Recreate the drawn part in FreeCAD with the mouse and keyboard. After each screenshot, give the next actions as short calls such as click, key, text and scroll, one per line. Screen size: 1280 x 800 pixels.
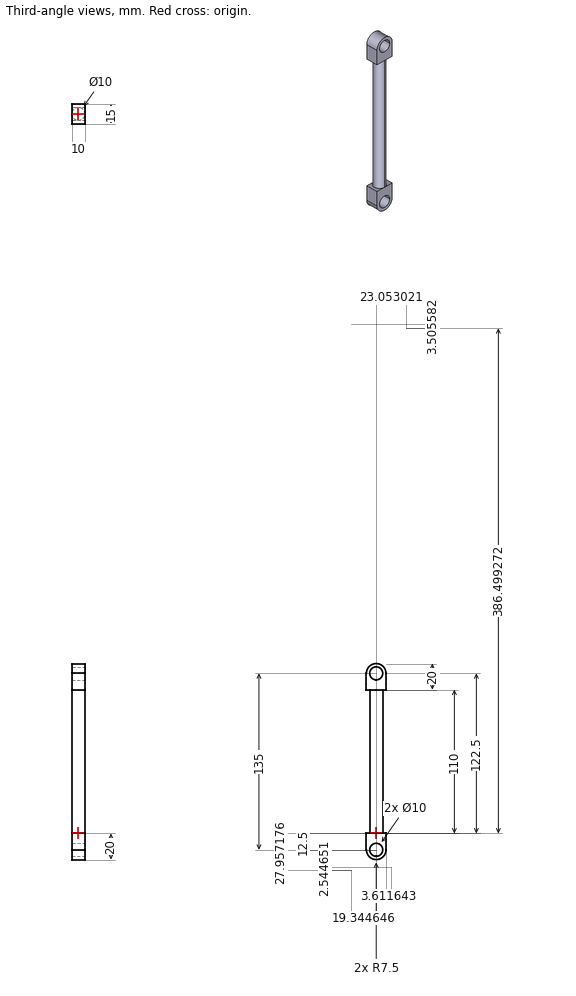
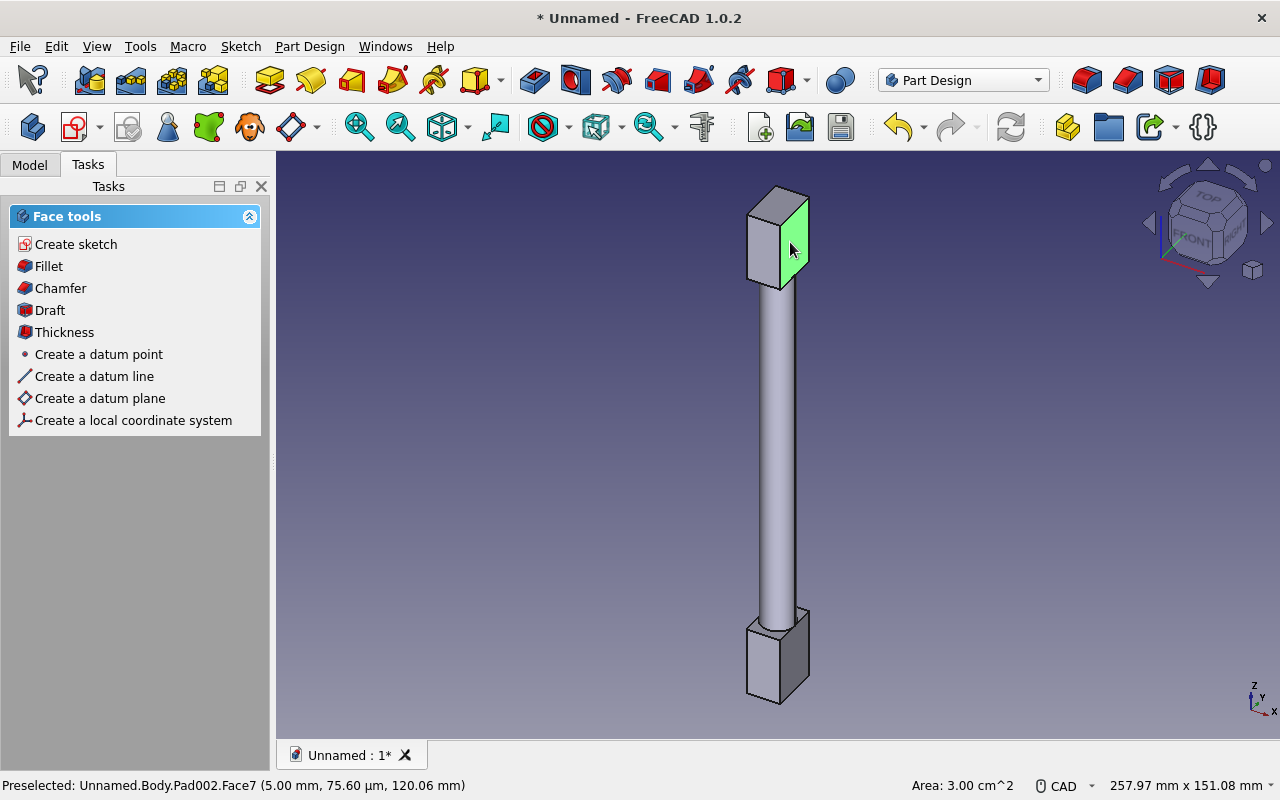
click(74, 128)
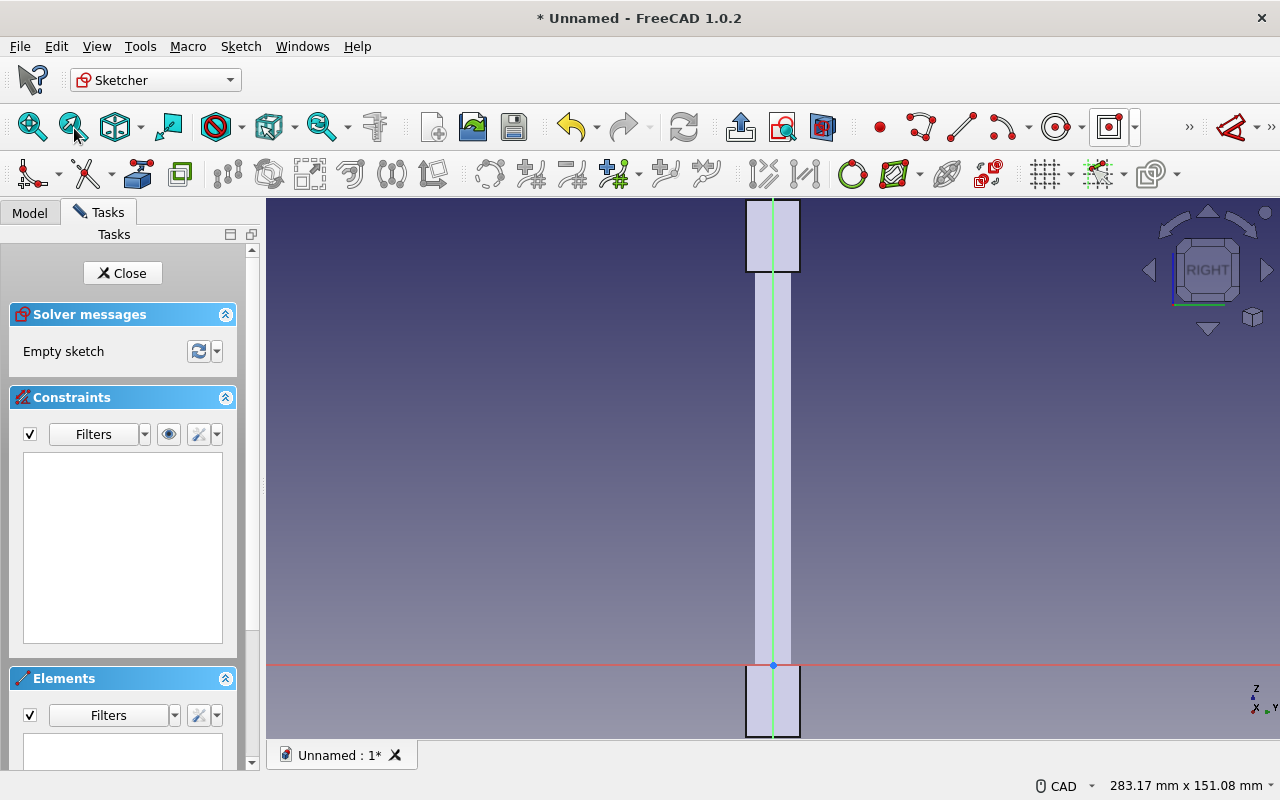
scroll(680, 616, down, 7)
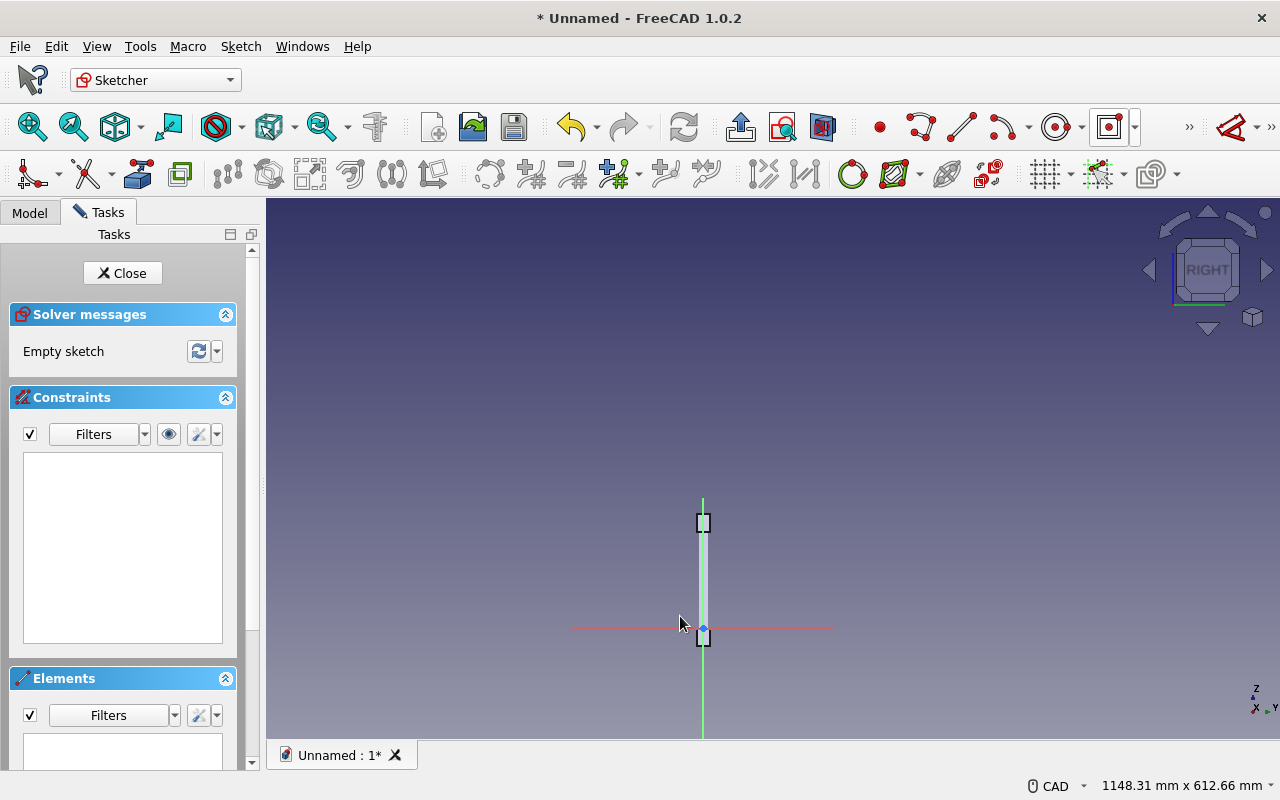
click(921, 128)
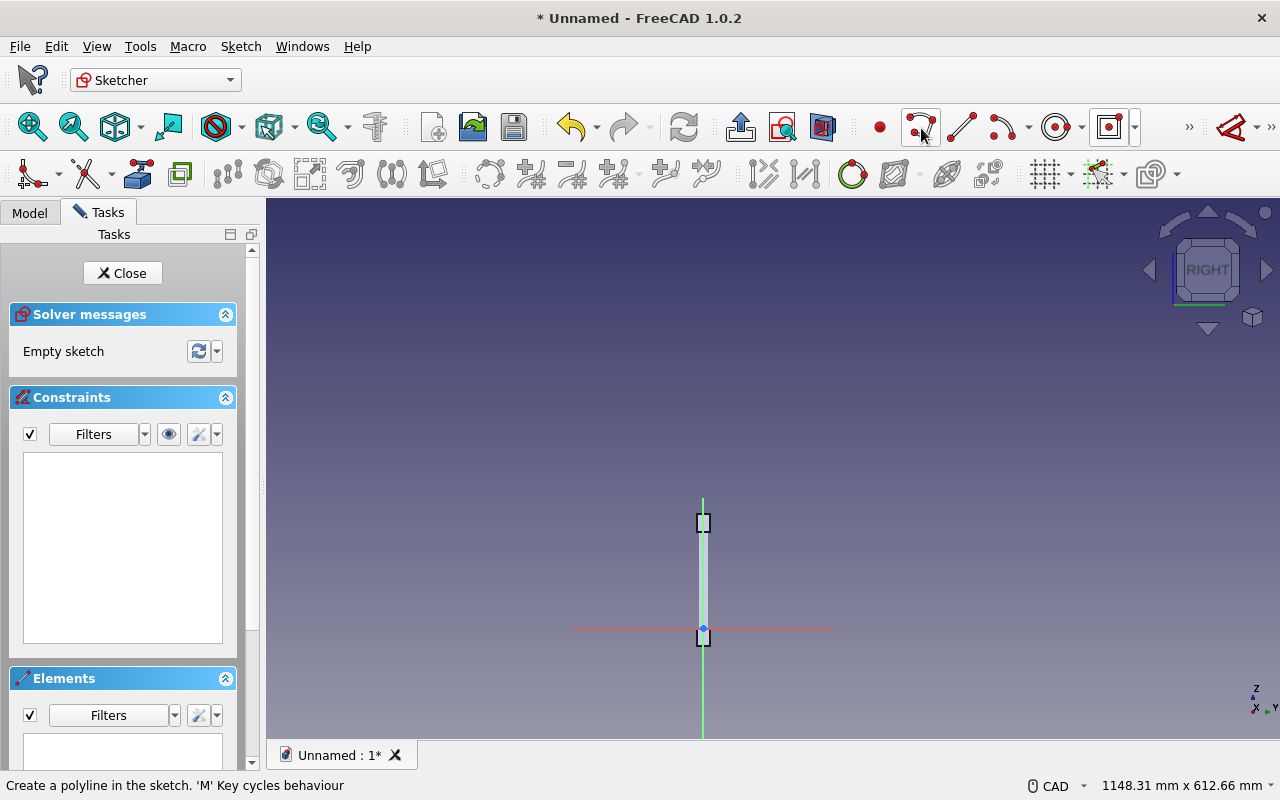
scroll(697, 640, up, 5)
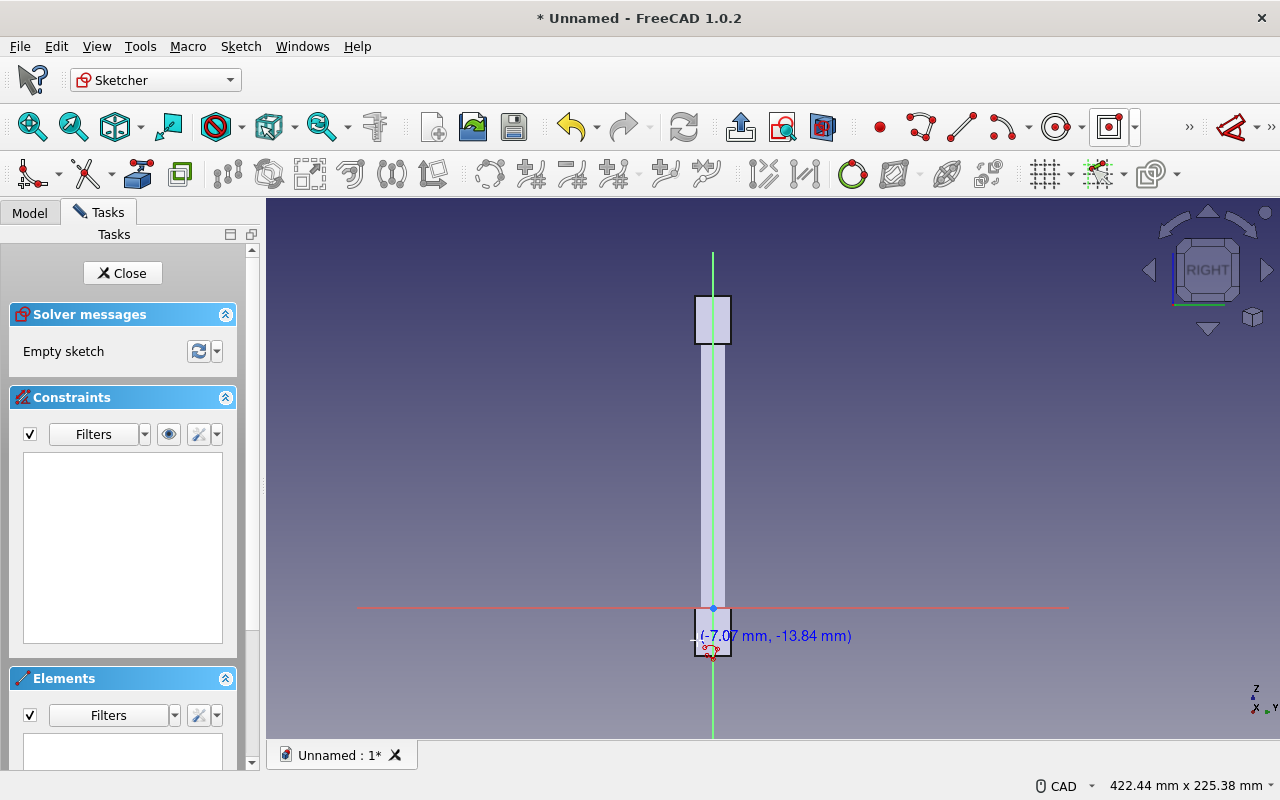
click(695, 638)
click(667, 675)
click(740, 669)
click(731, 638)
right_click(731, 638)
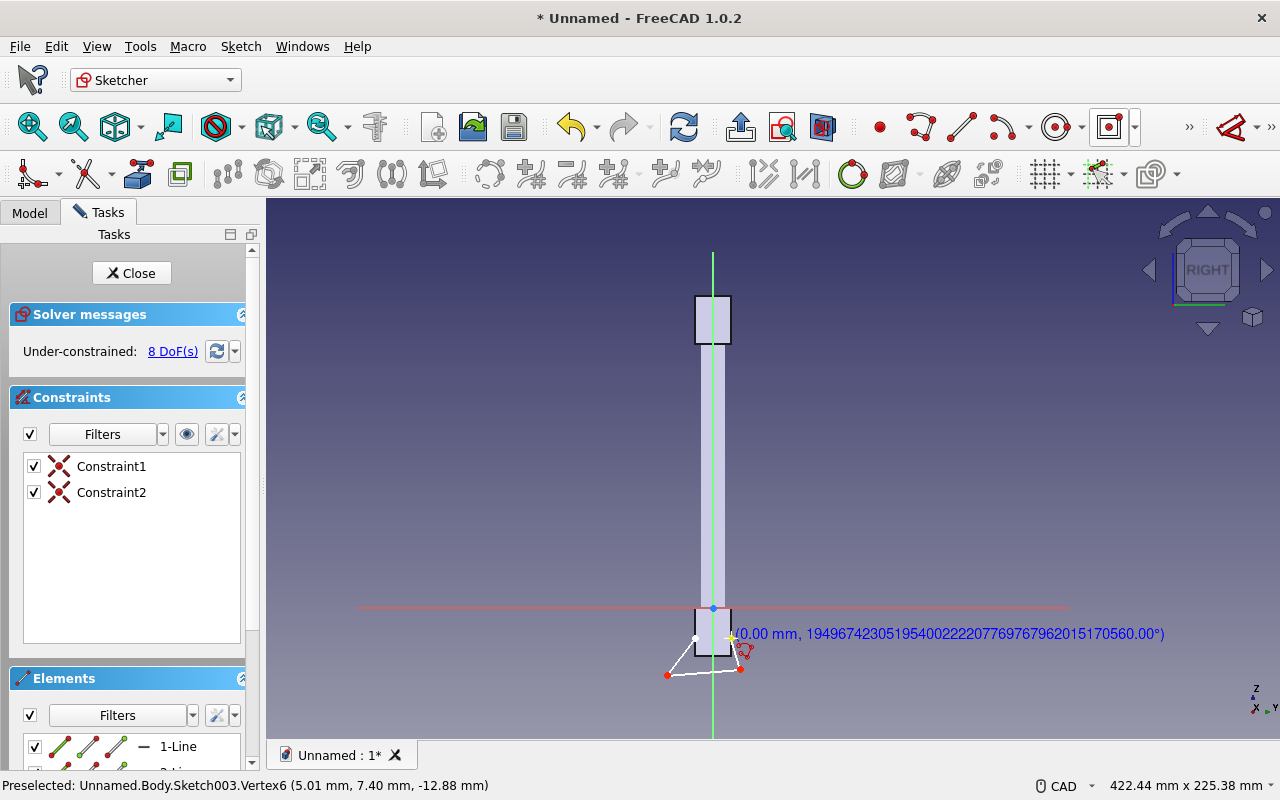
click(1028, 128)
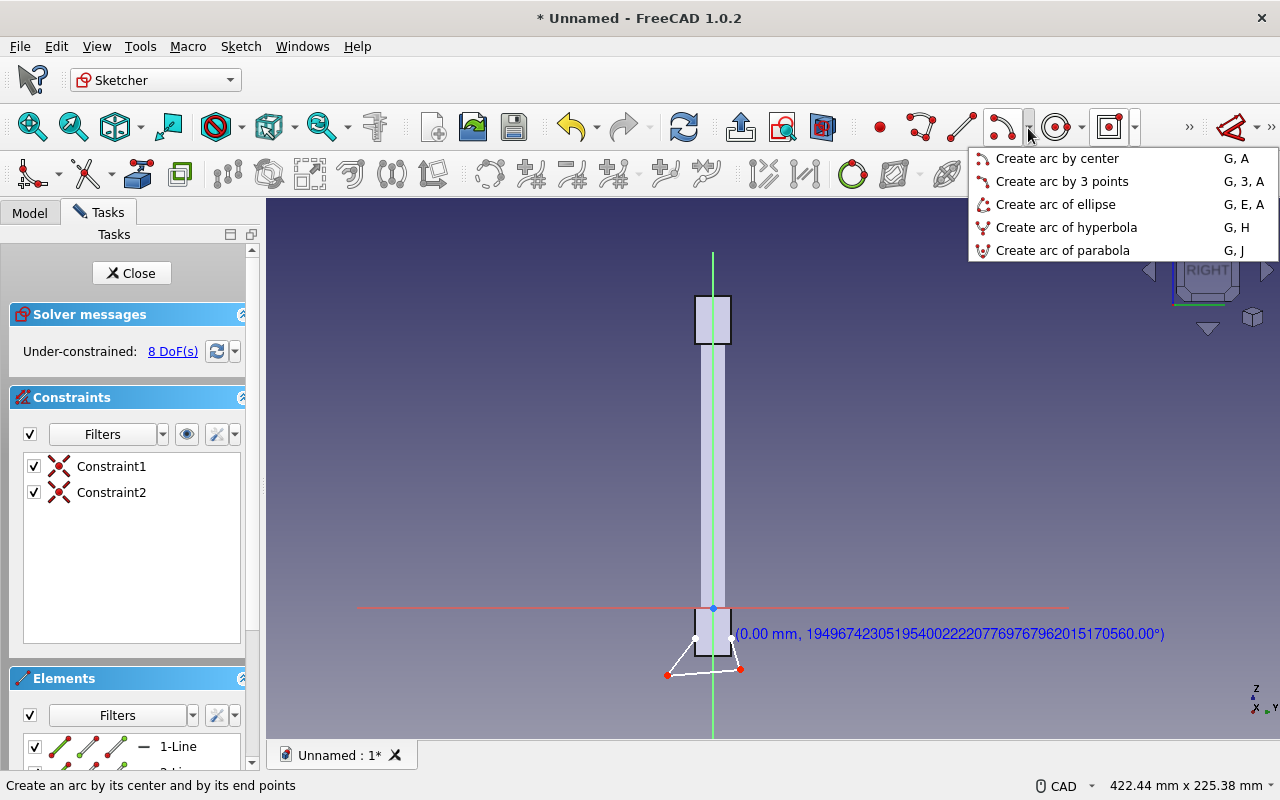
click(1124, 182)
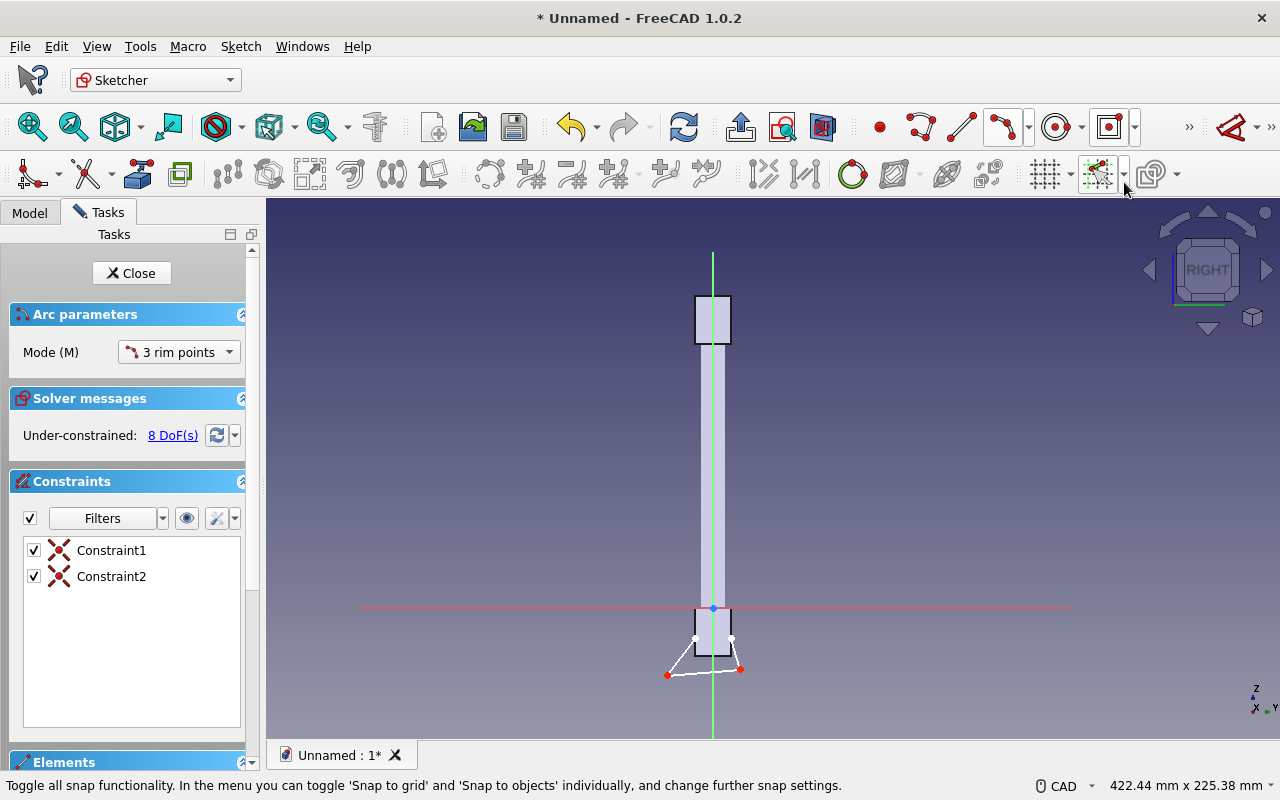
click(731, 639)
click(695, 639)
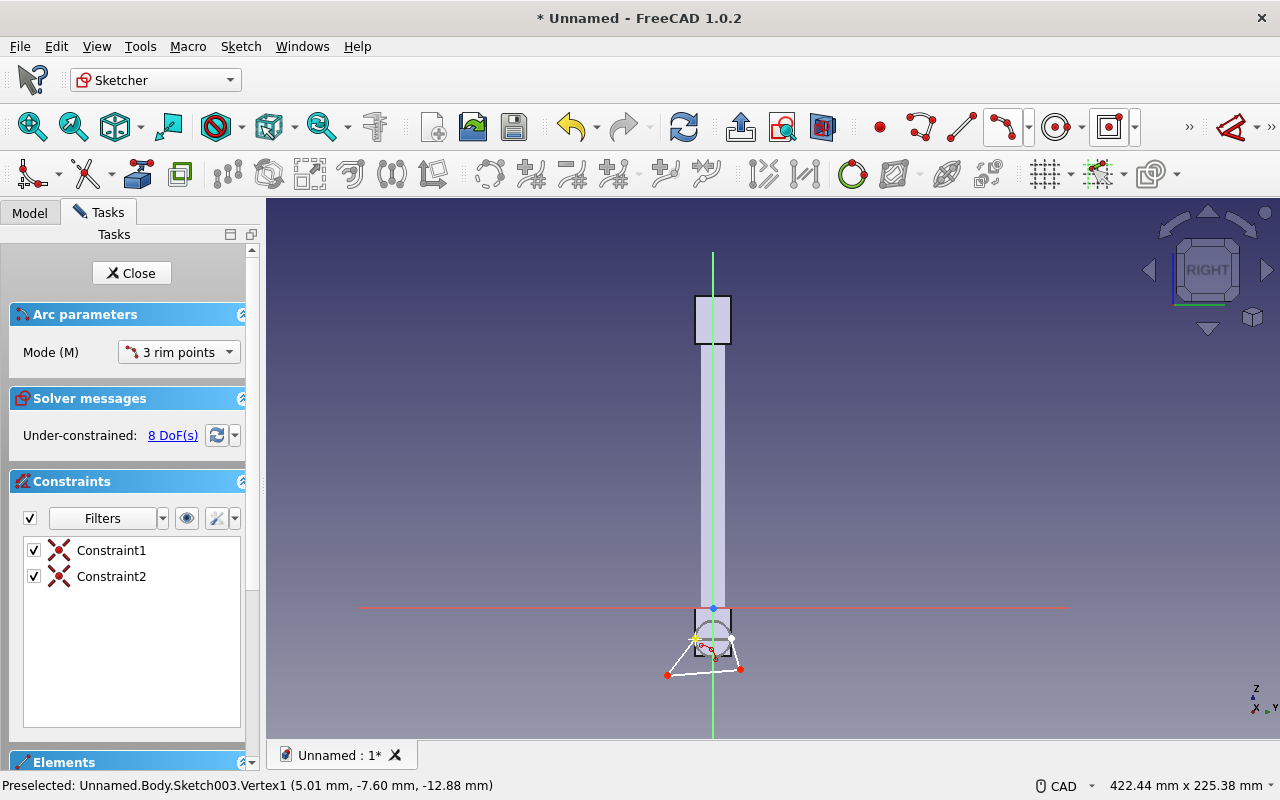
scroll(703, 653, up, 3)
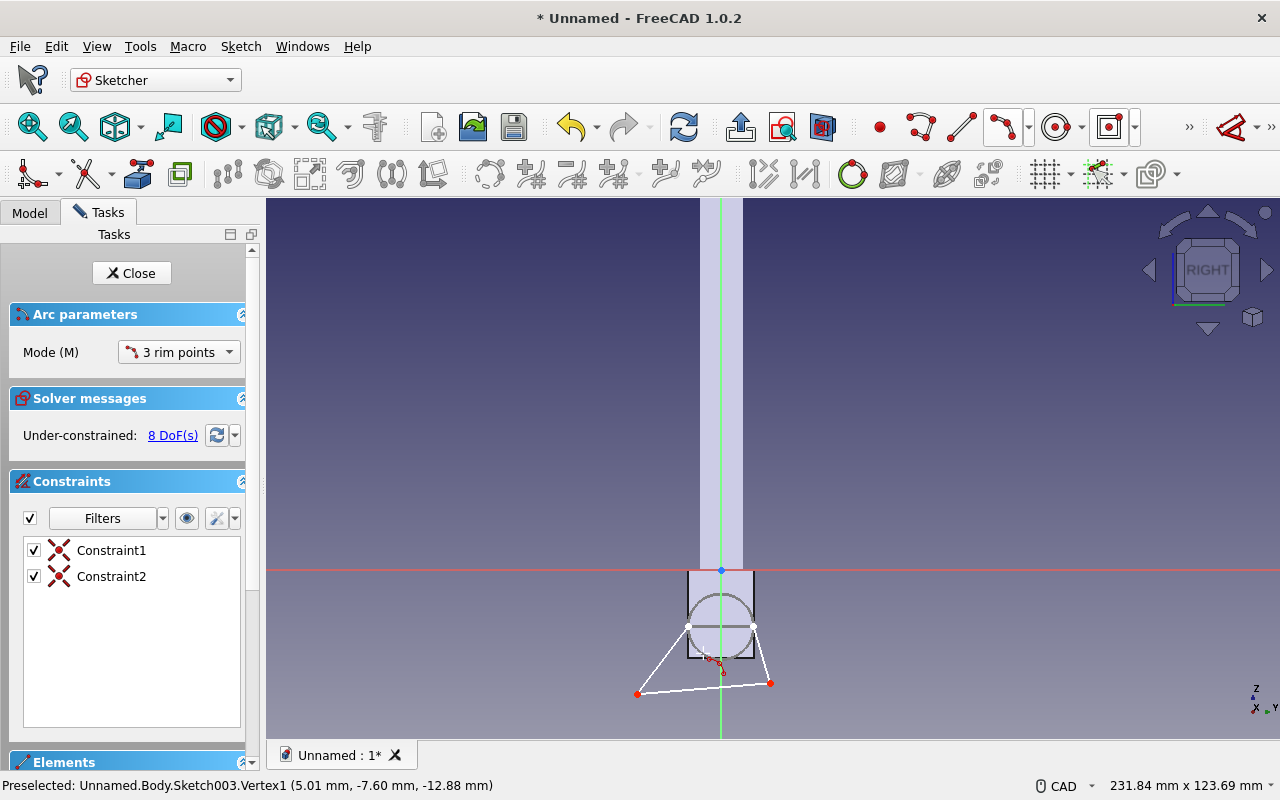
click(702, 652)